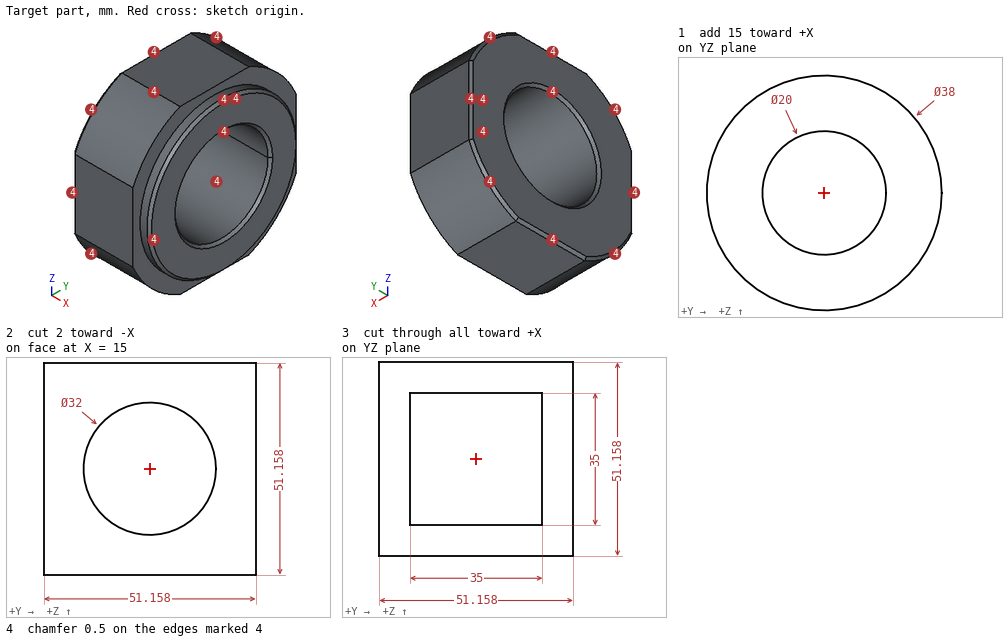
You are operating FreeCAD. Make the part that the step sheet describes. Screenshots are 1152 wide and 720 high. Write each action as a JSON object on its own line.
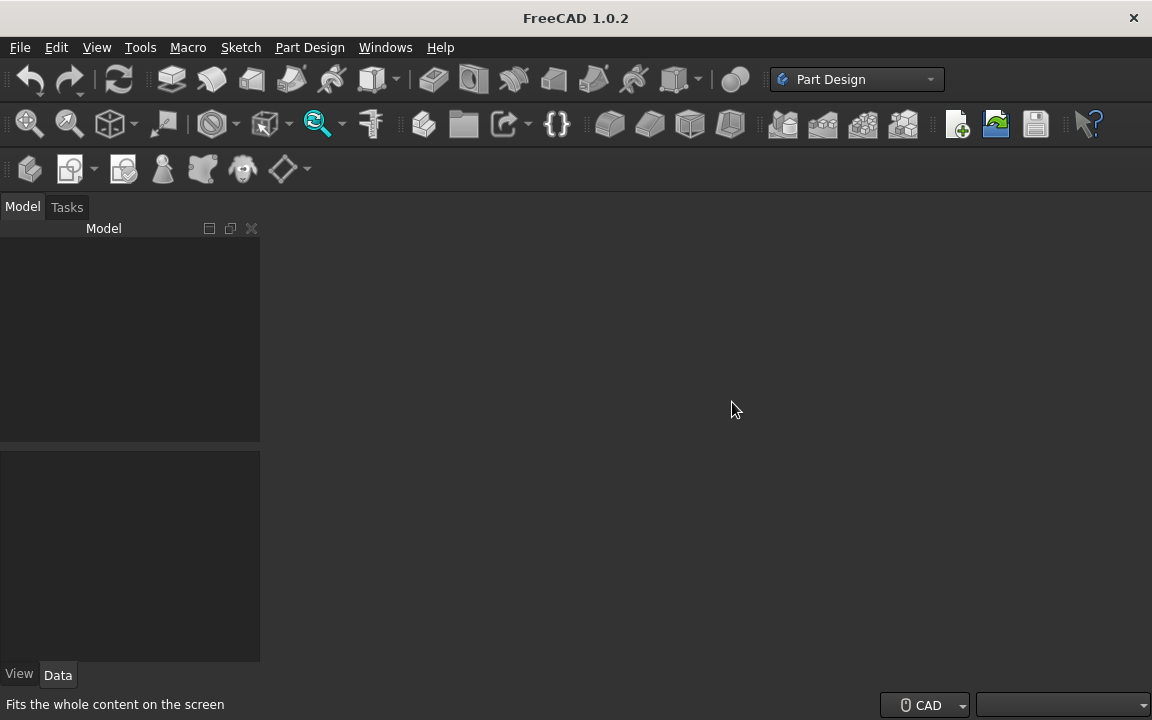
{"action": "key", "text": "ctrl+n"}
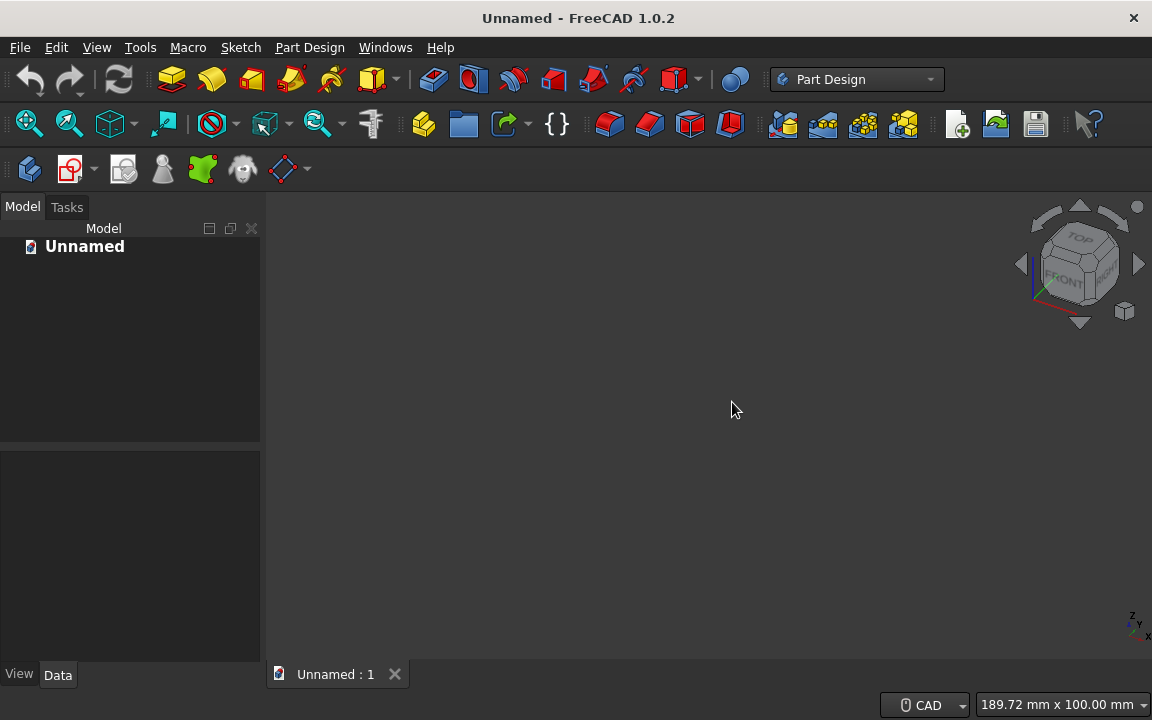
{"action": "left_click", "coordinate": [70, 170]}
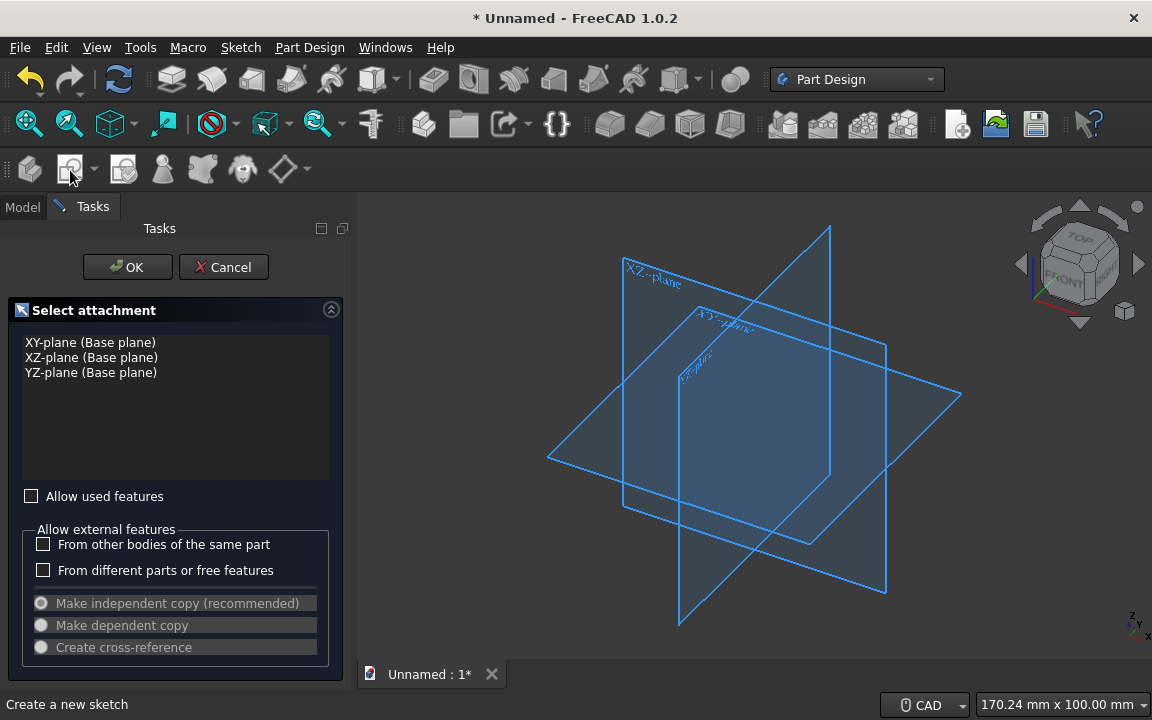
{"action": "left_click", "coordinate": [82, 372]}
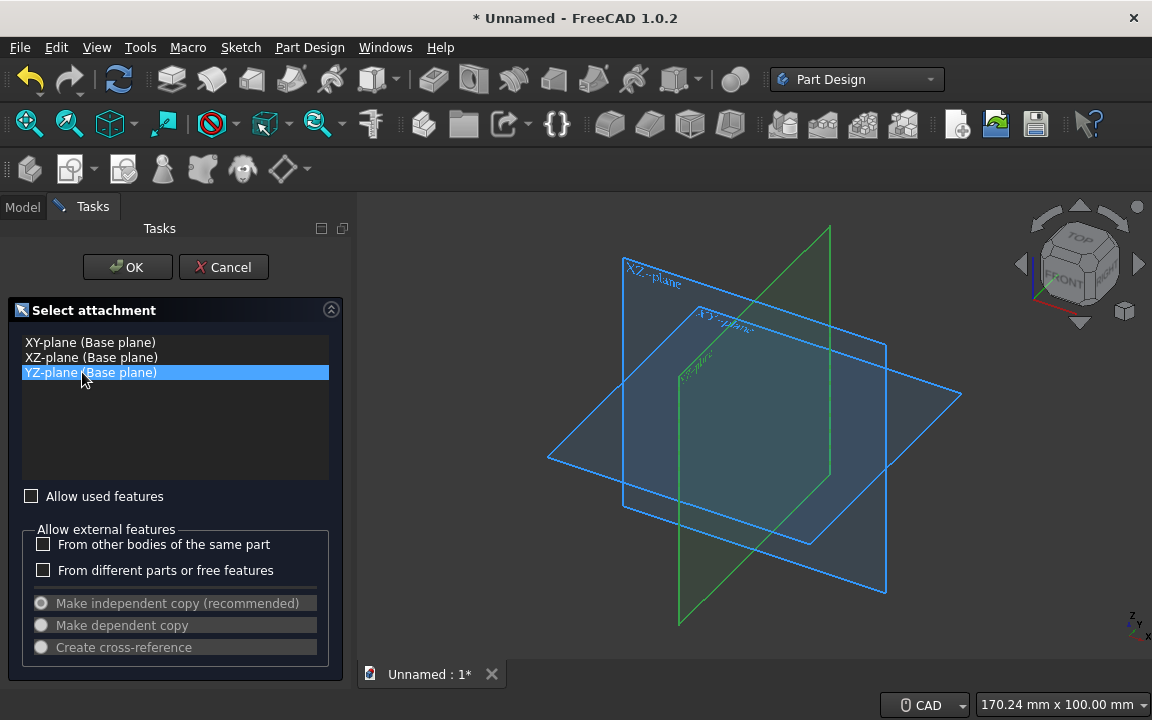
{"action": "left_click", "coordinate": [128, 267]}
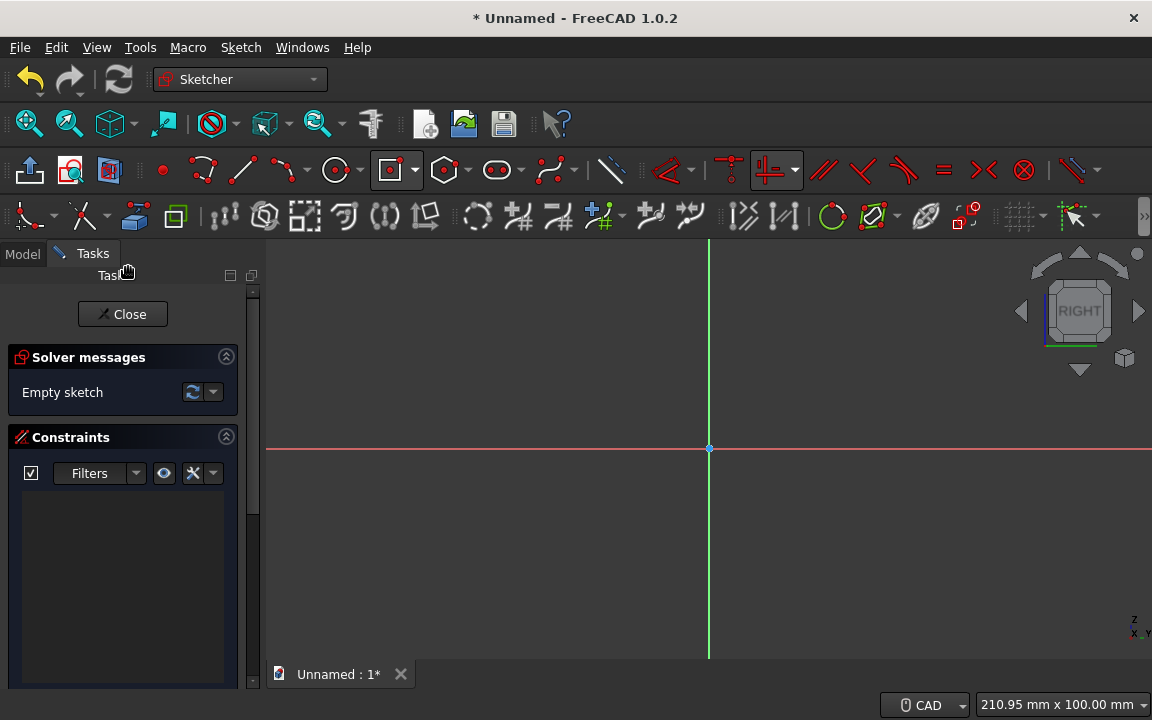
{"action": "scroll", "coordinate": [848, 449], "scroll_direction": "up", "scroll_amount": 2}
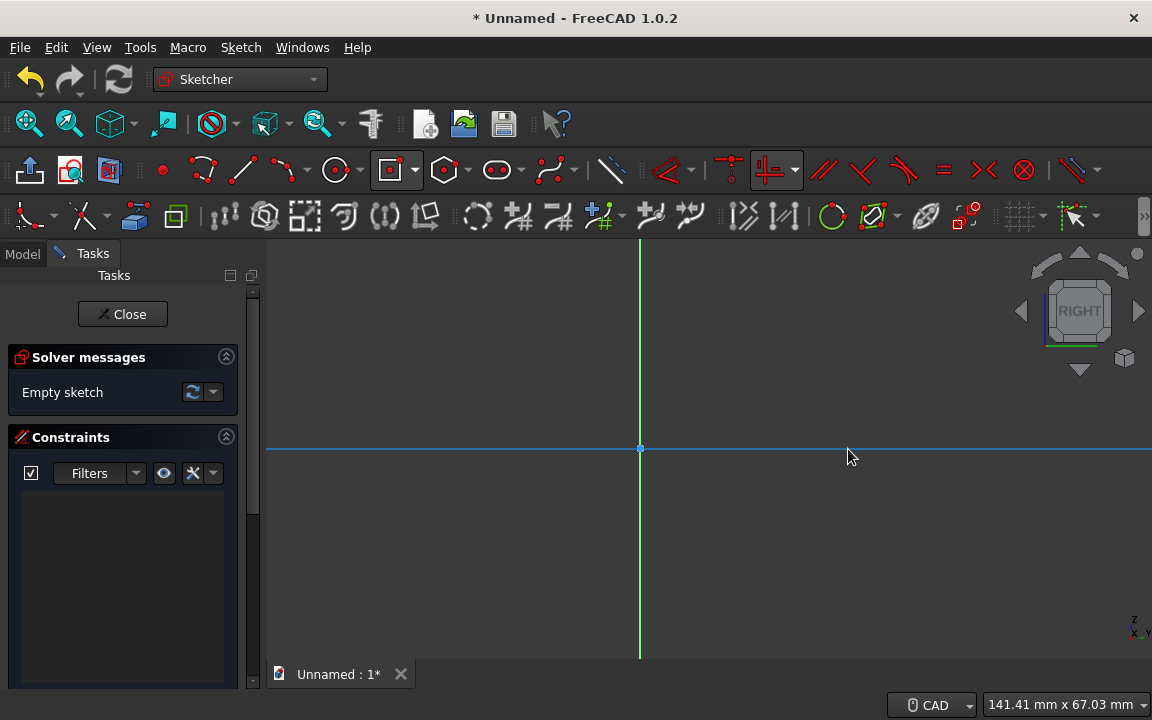
{"action": "key", "text": "g c"}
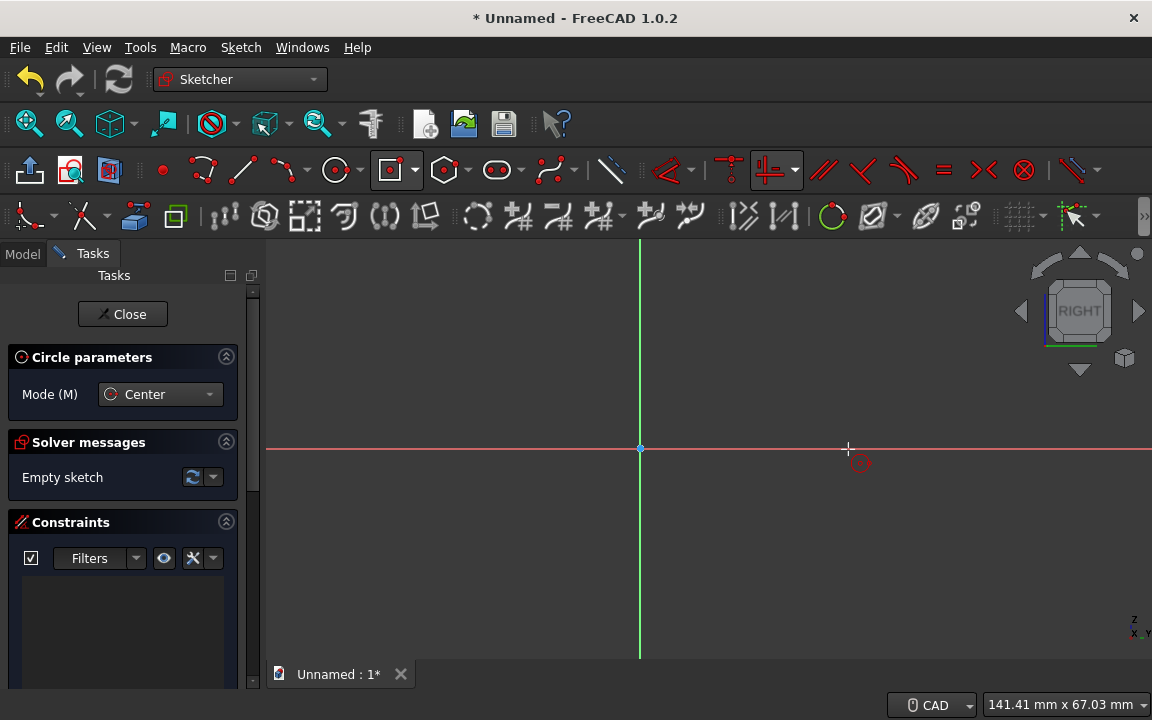
{"action": "left_click", "coordinate": [640, 449]}
{"action": "left_click", "coordinate": [724, 365]}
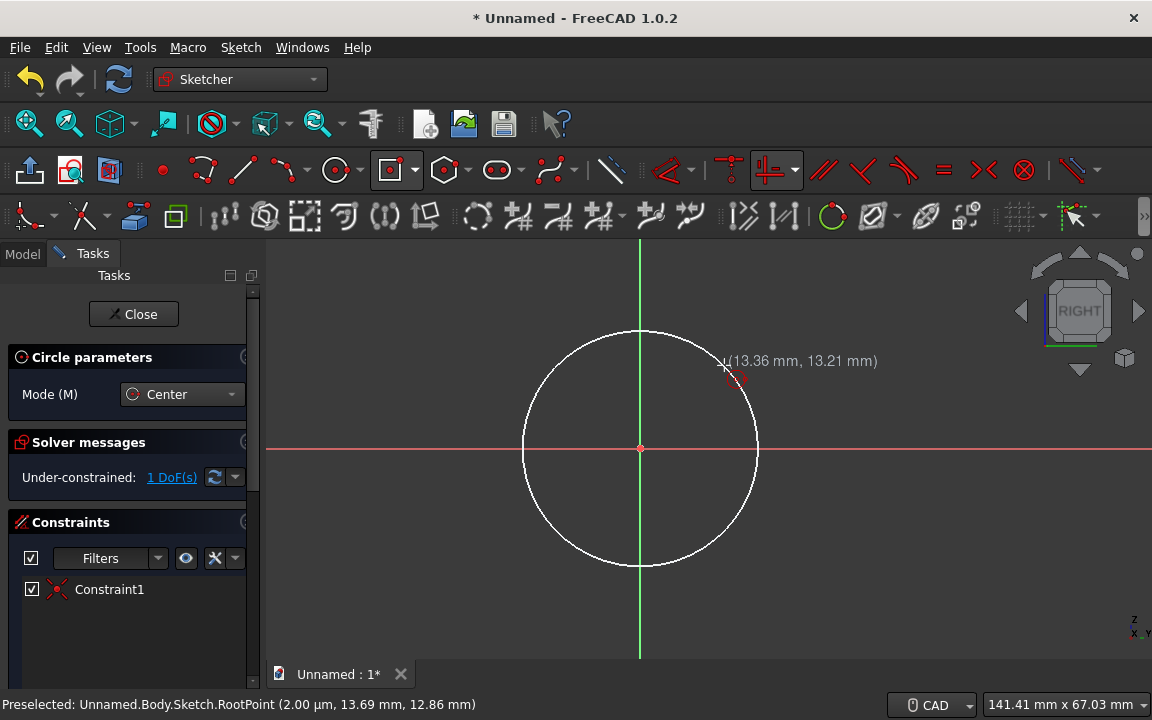
{"action": "left_click", "coordinate": [640, 449]}
{"action": "left_click", "coordinate": [685, 404]}
{"action": "key", "text": "Escape"}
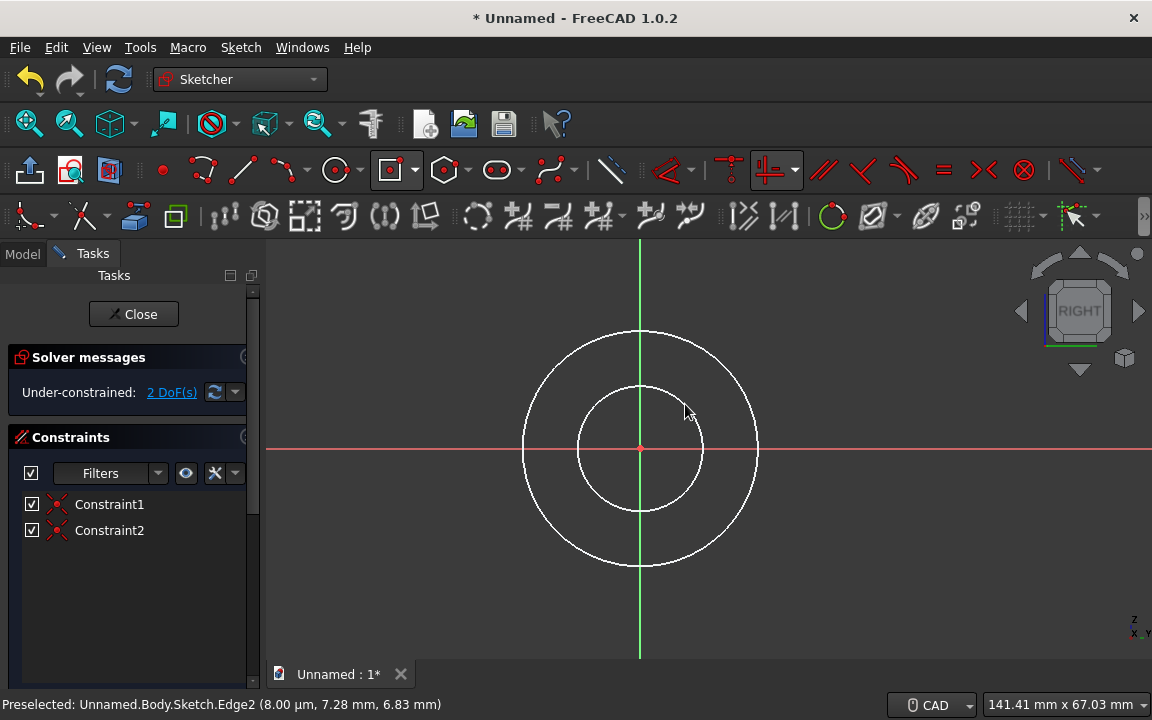
{"action": "key", "text": "d"}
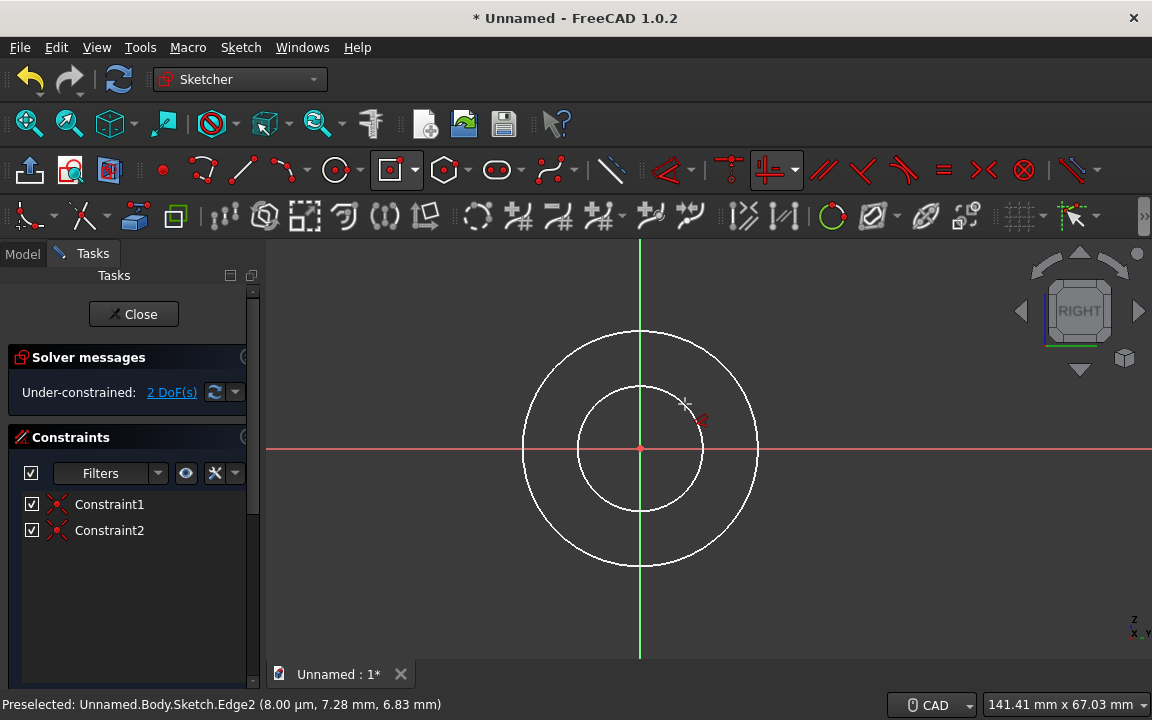
{"action": "left_click", "coordinate": [723, 365]}
{"action": "left_click", "coordinate": [745, 342]}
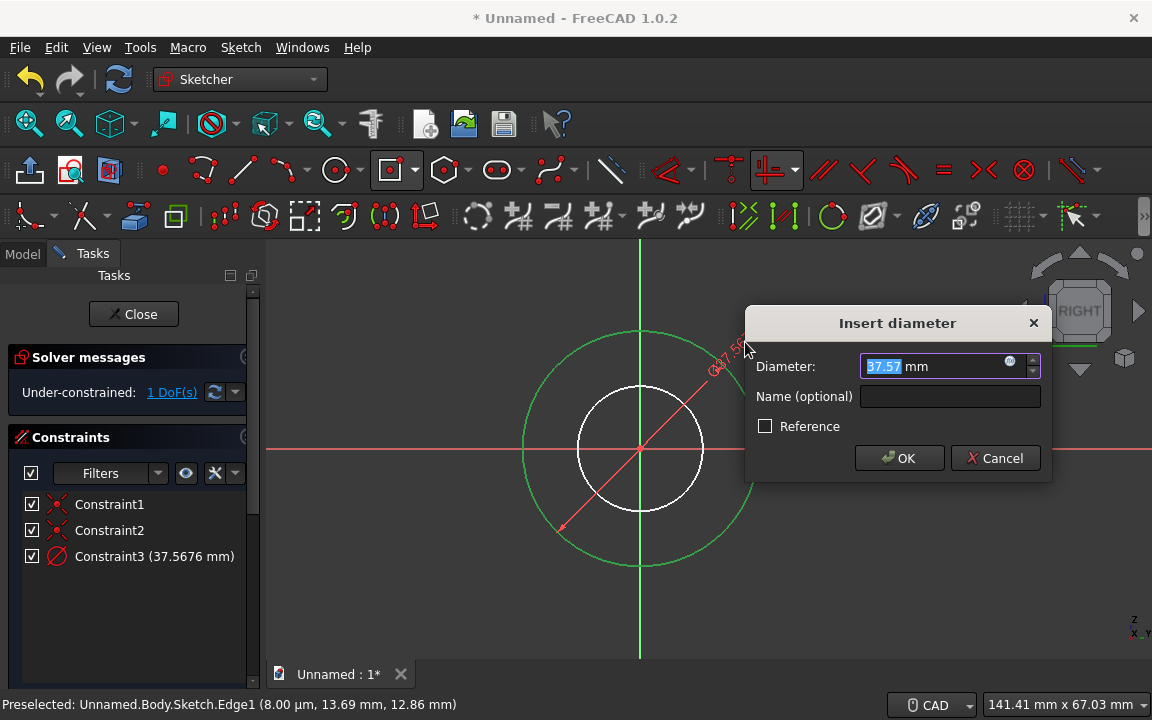
{"action": "type", "text": "38"}
{"action": "key", "text": "Return"}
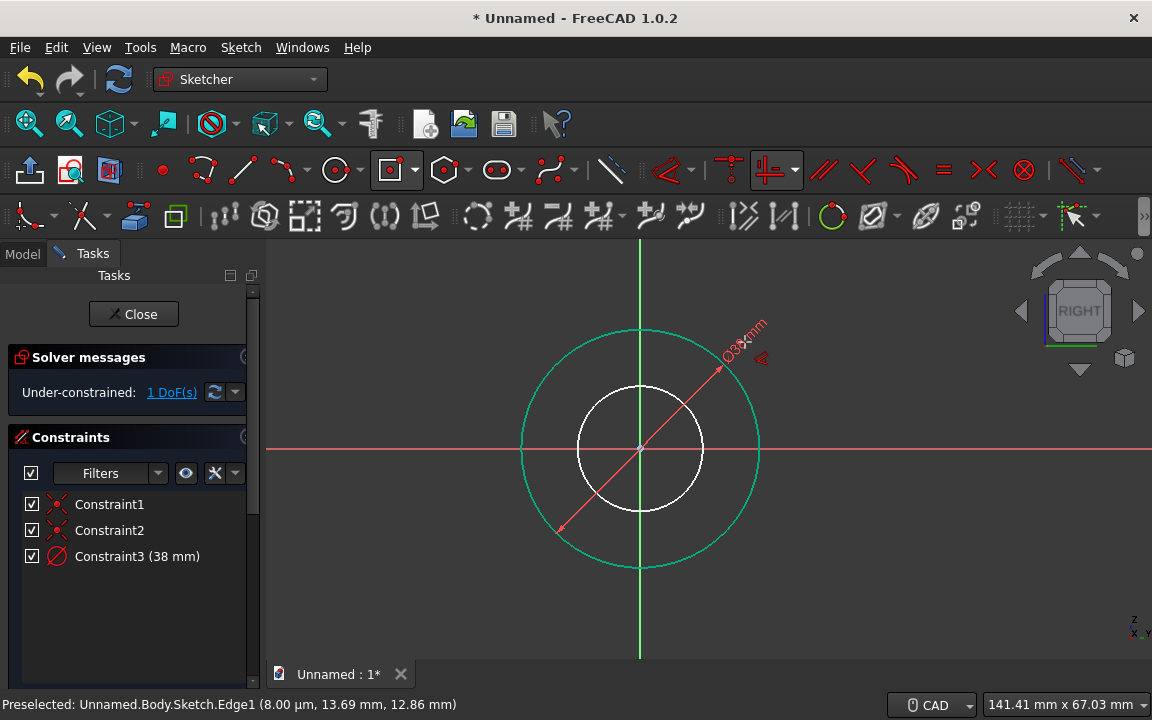
{"action": "left_click", "coordinate": [684, 404]}
{"action": "left_click", "coordinate": [706, 381]}